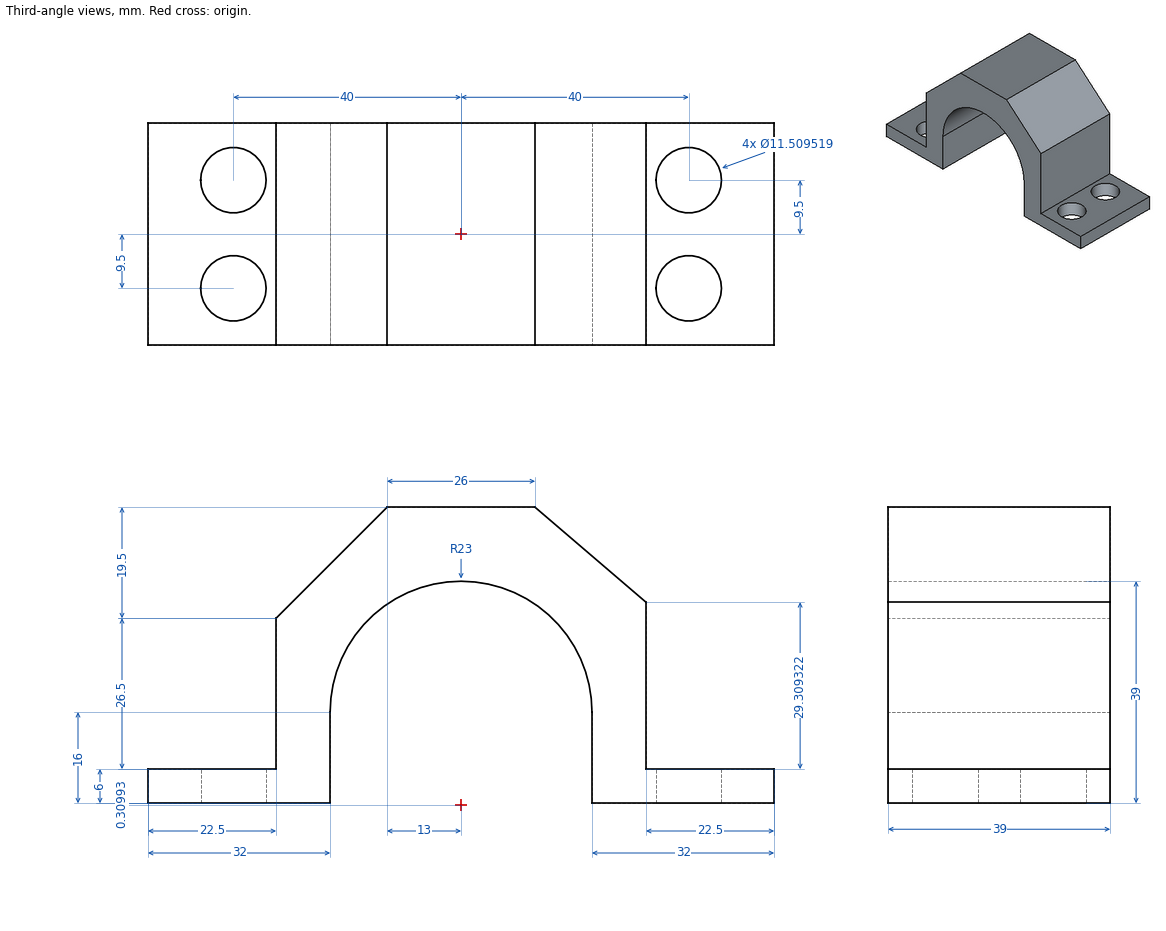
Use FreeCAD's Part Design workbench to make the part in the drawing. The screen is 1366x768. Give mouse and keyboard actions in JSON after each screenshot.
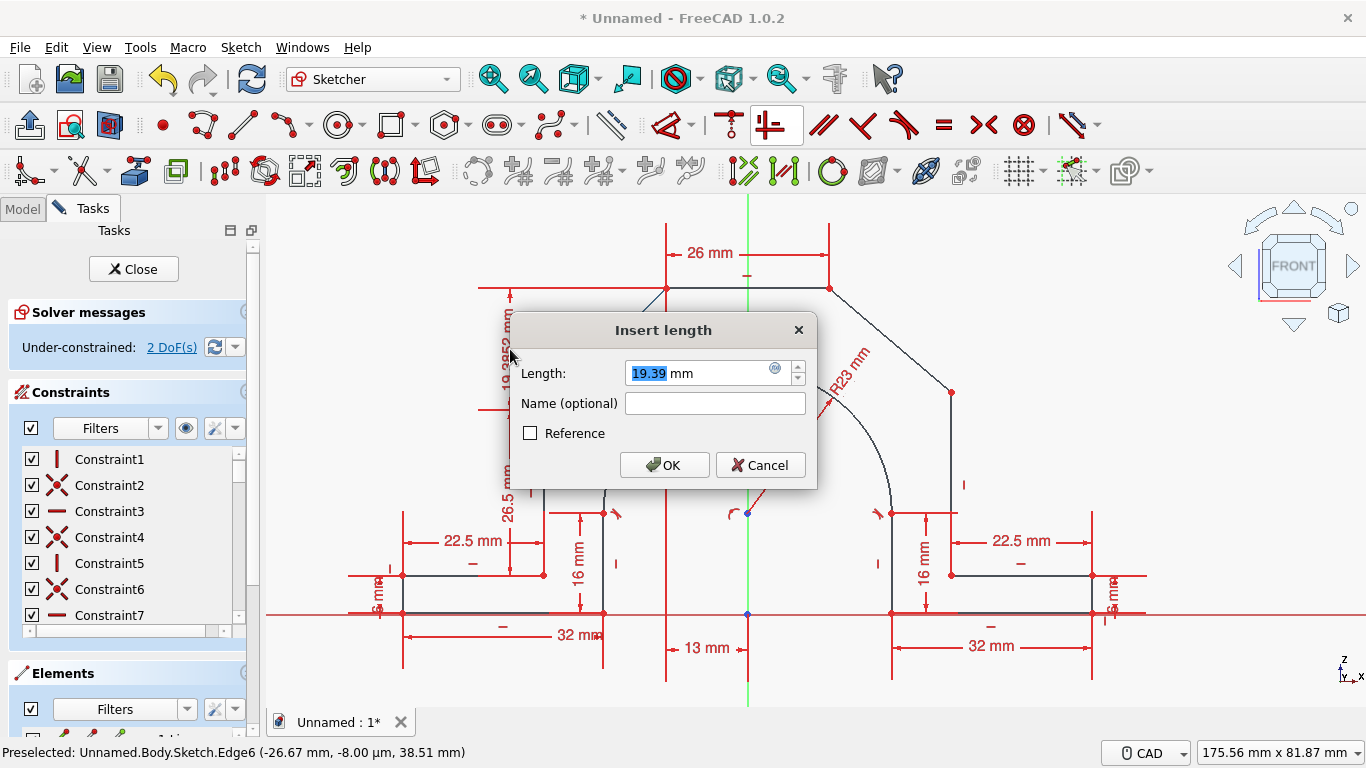
{"action": "type", "text": "19.5"}
{"action": "key", "text": "Return"}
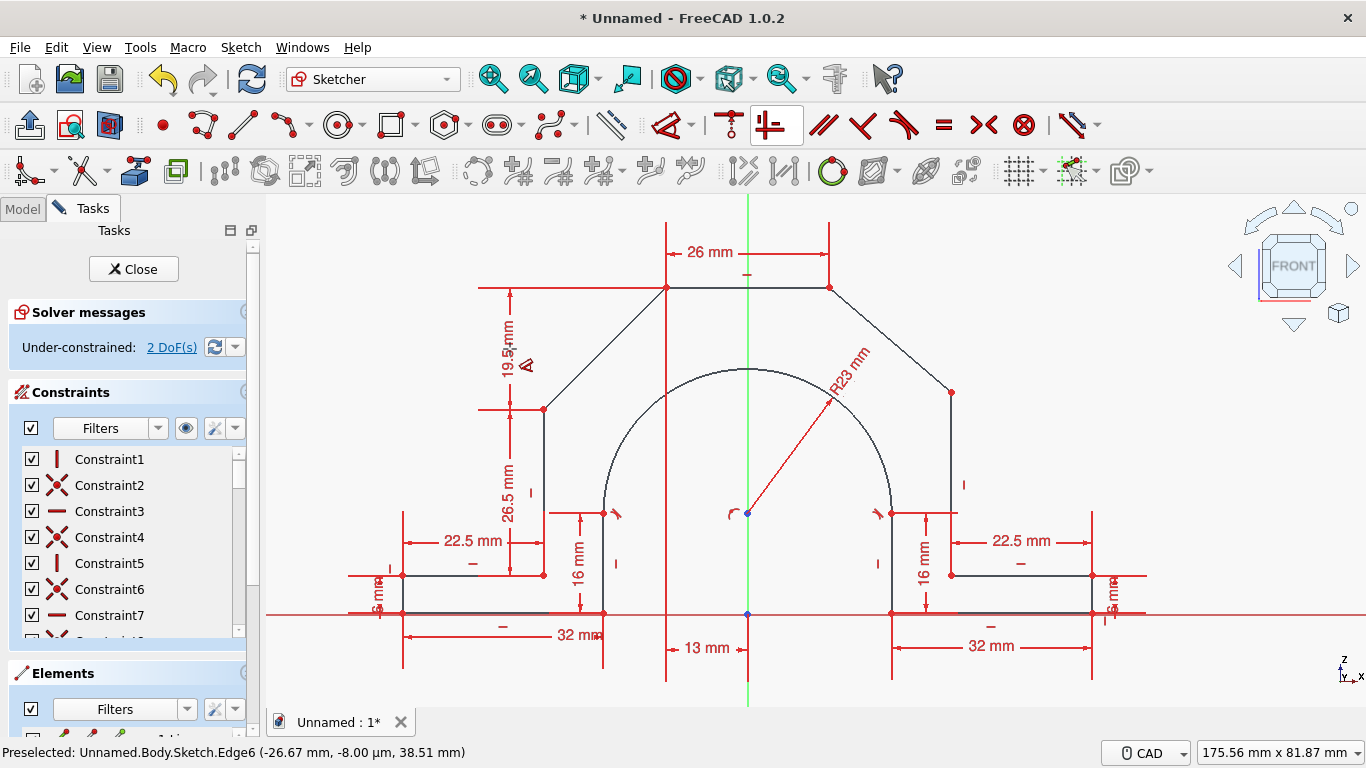
{"action": "scroll", "coordinate": [603, 613], "scroll_direction": "up", "scroll_amount": 16}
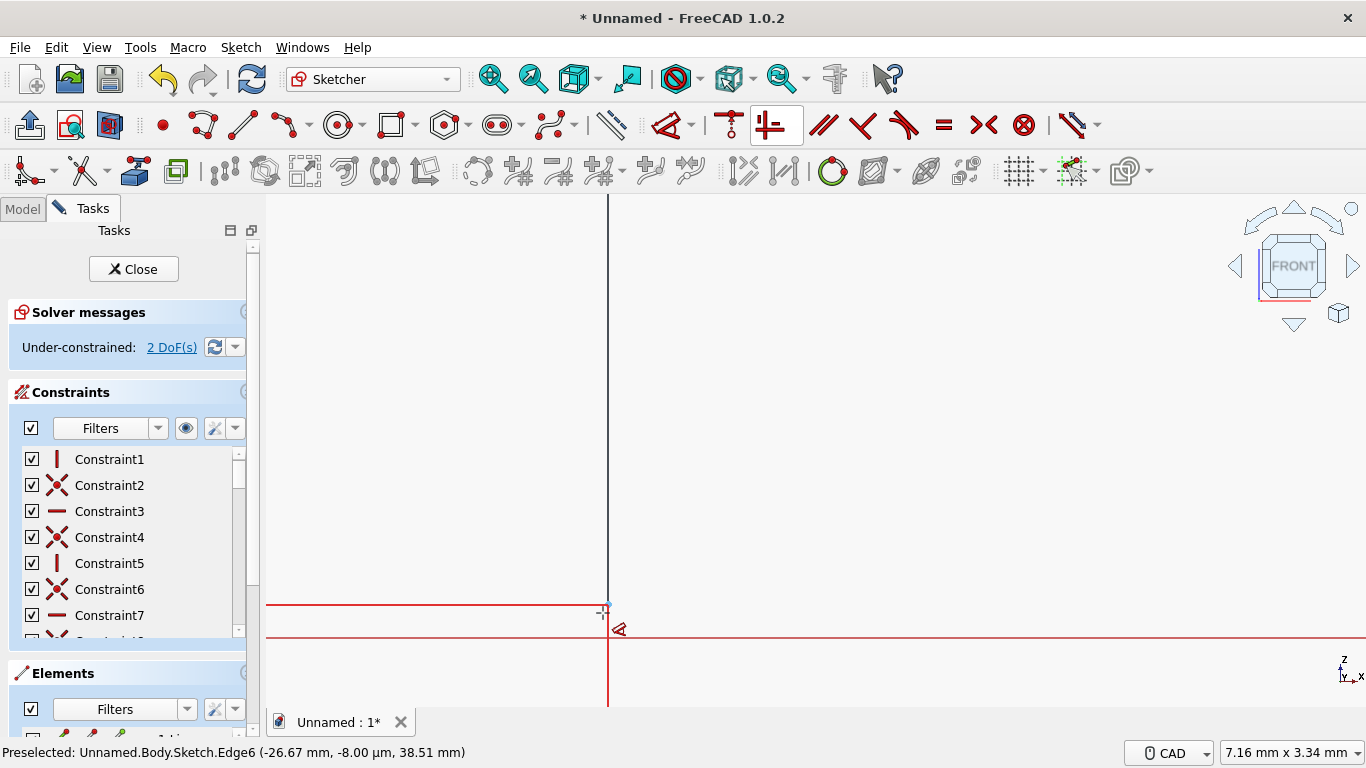
{"action": "left_click", "coordinate": [608, 605]}
{"action": "left_click", "coordinate": [574, 621]}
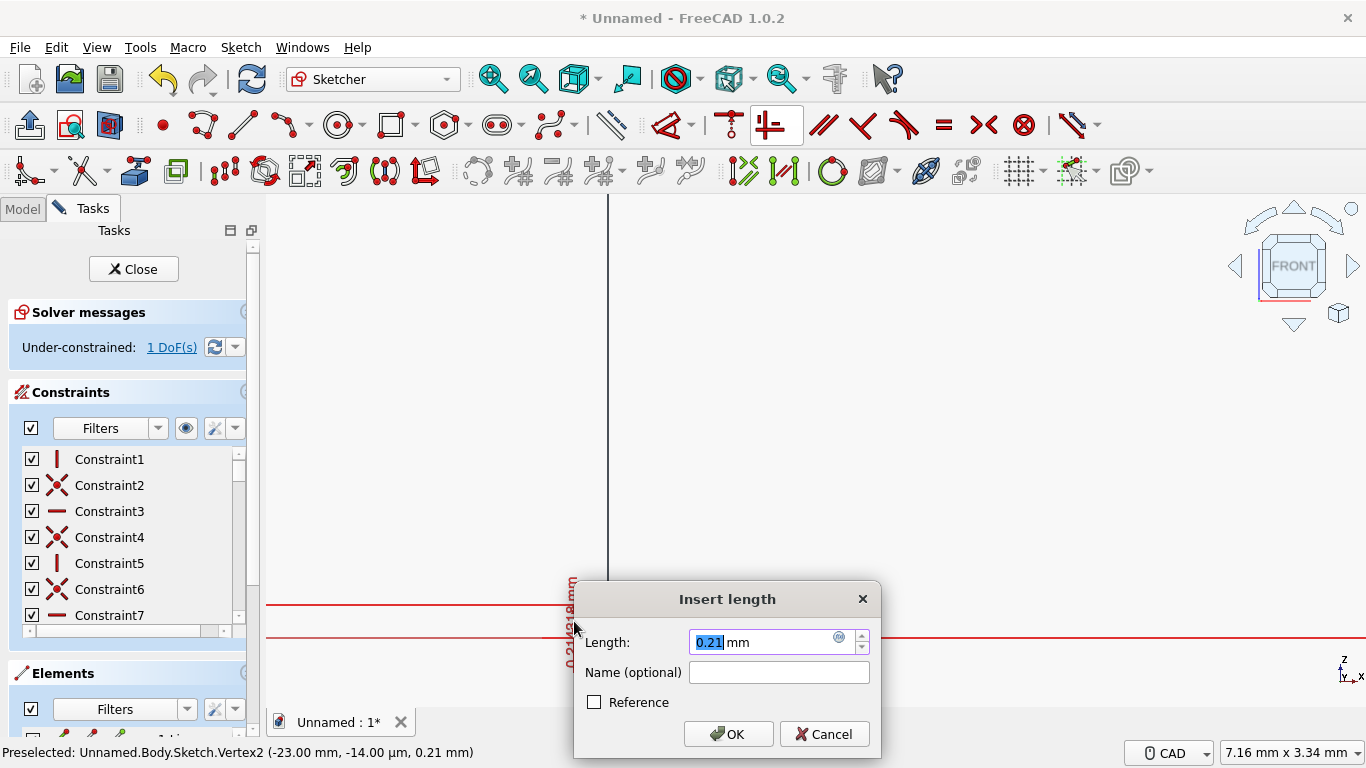
{"action": "type", "text": "0.30993"}
{"action": "key", "text": "Return"}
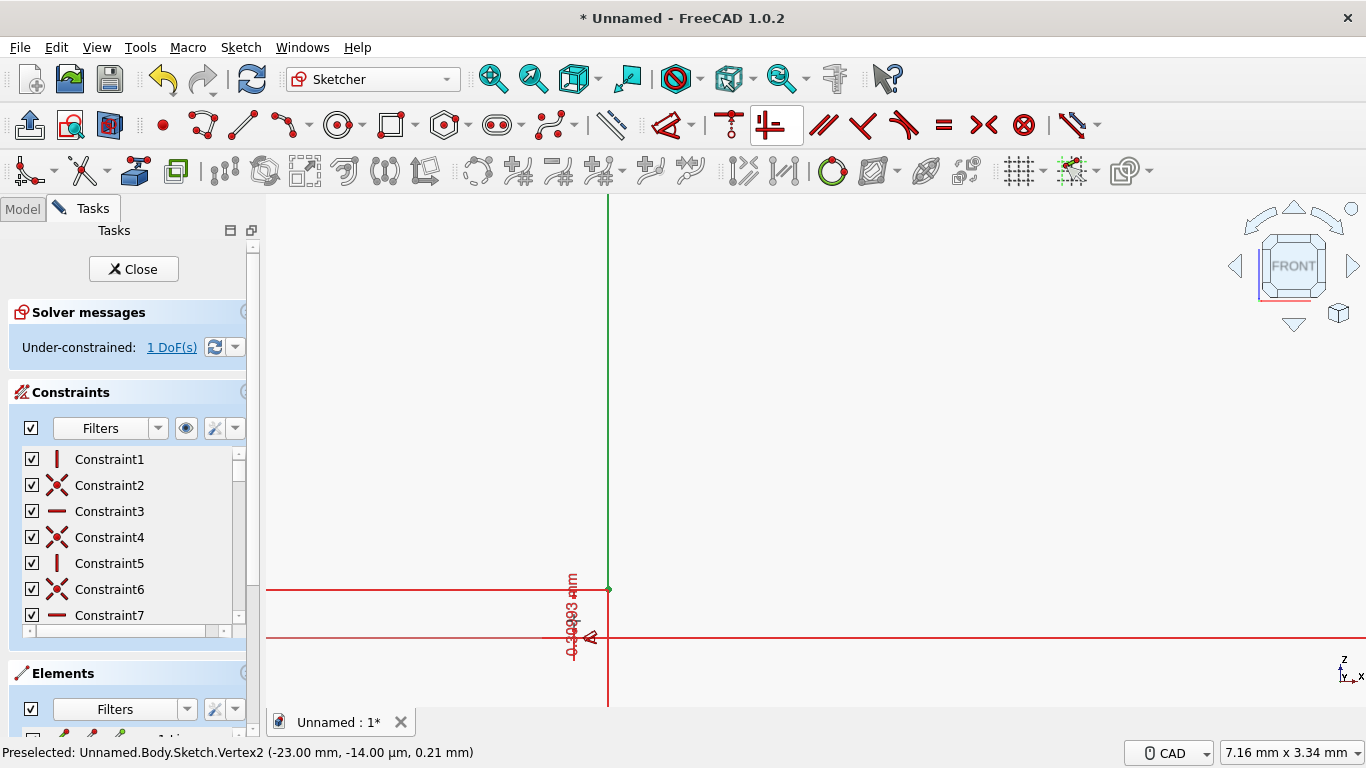
{"action": "scroll", "coordinate": [570, 651], "scroll_direction": "down", "scroll_amount": 15}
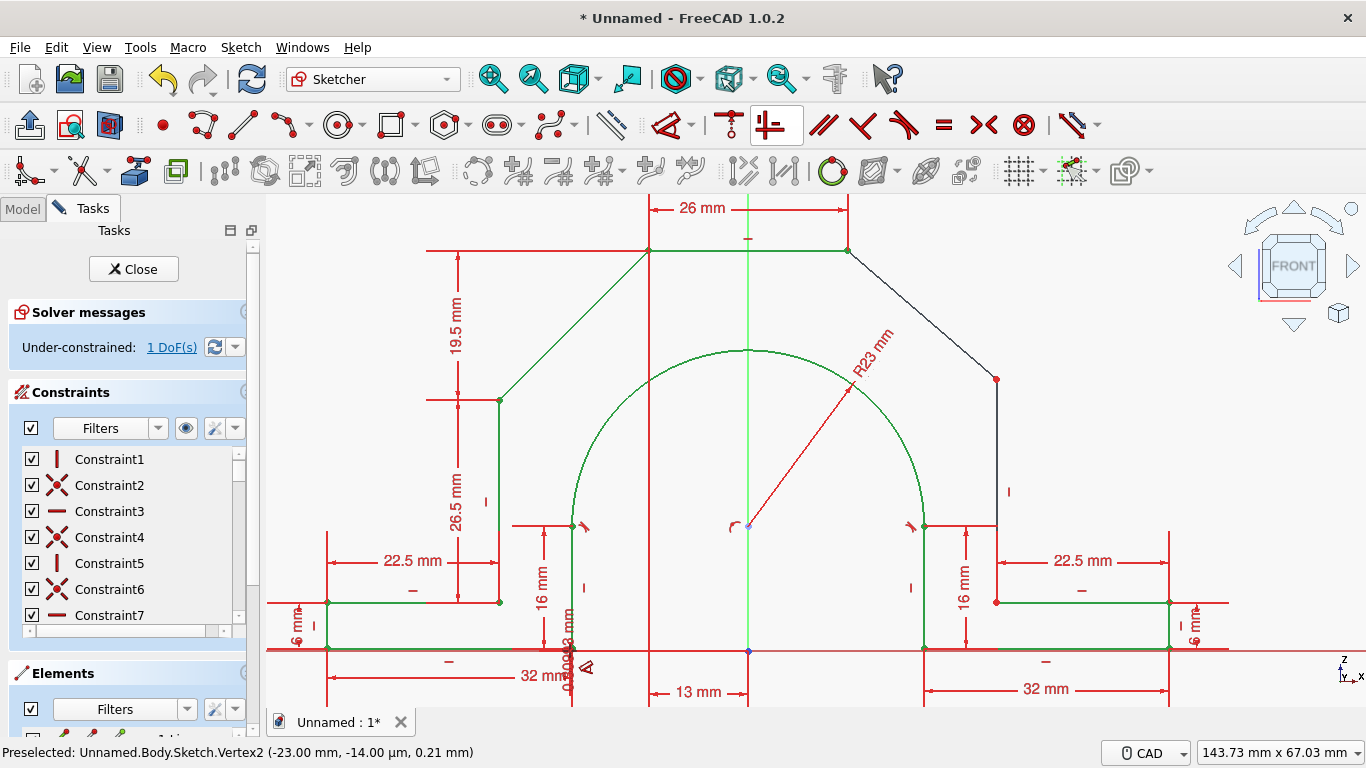
{"action": "left_click", "coordinate": [997, 447]}
{"action": "left_click", "coordinate": [1031, 491]}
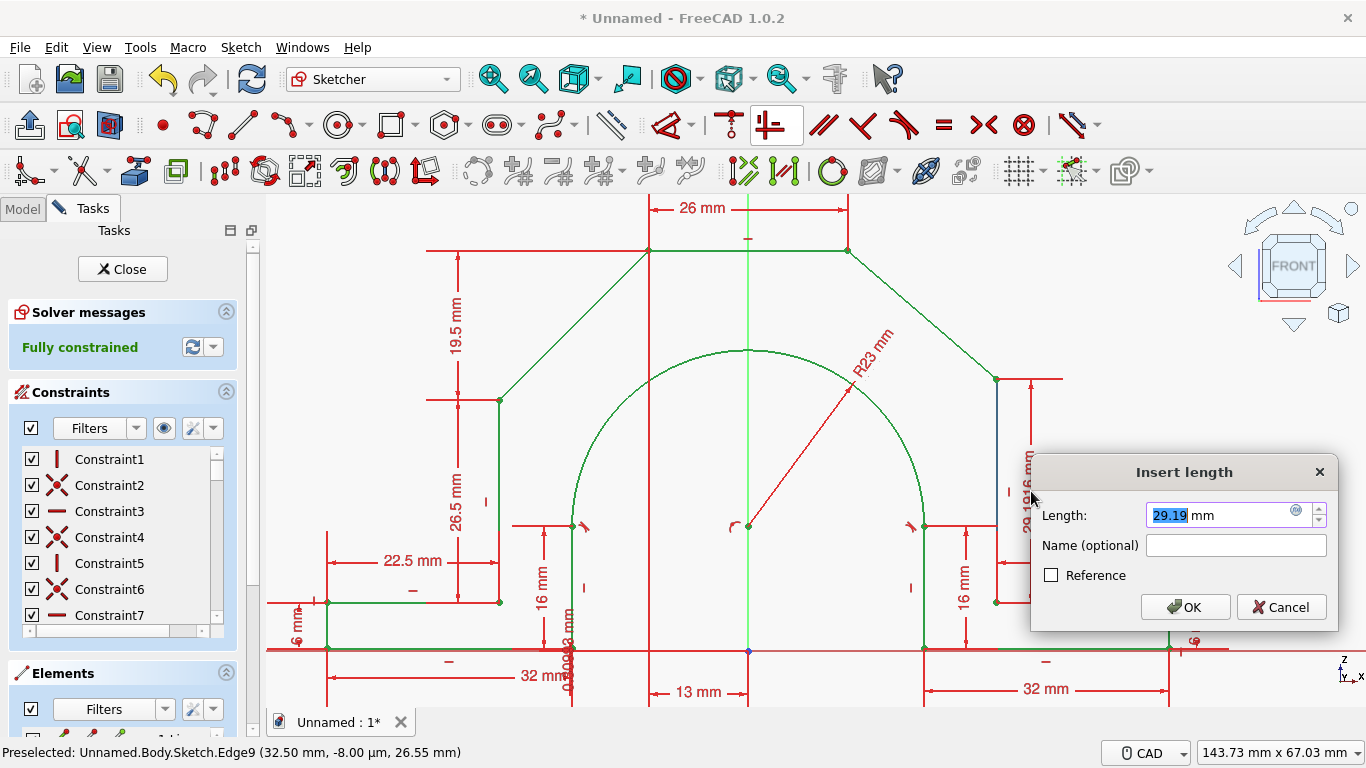
{"action": "type", "text": "29.309322"}
{"action": "key", "text": "Return"}
{"action": "key", "text": "Escape"}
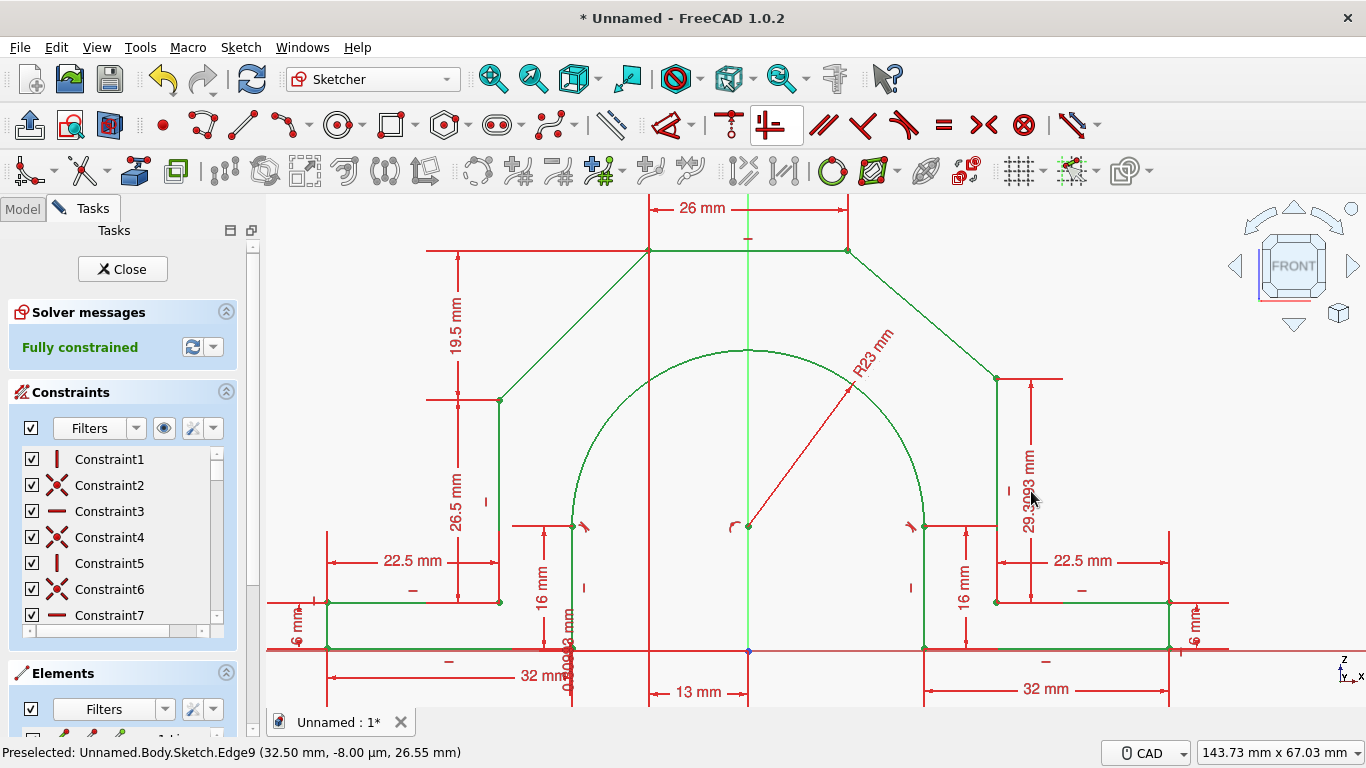
{"action": "left_click", "coordinate": [123, 269]}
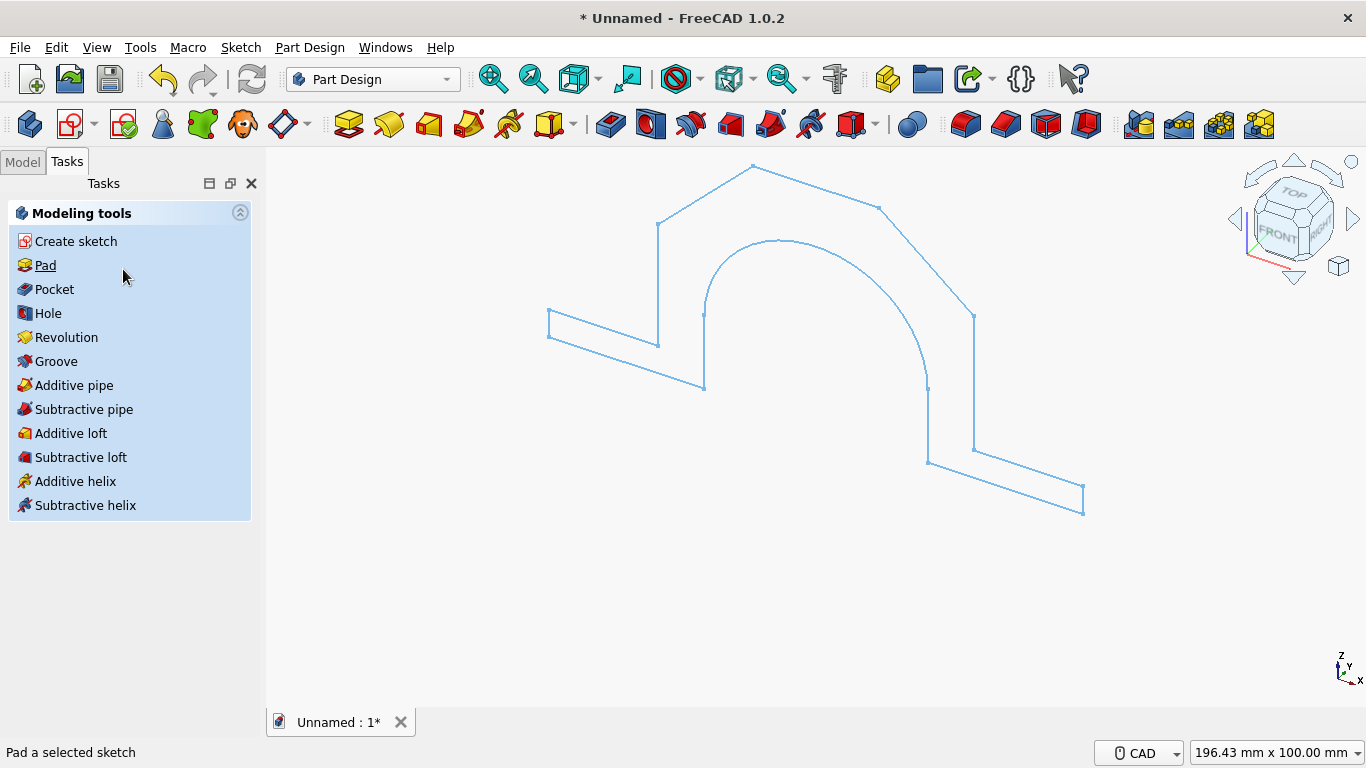
{"action": "left_click", "coordinate": [350, 124]}